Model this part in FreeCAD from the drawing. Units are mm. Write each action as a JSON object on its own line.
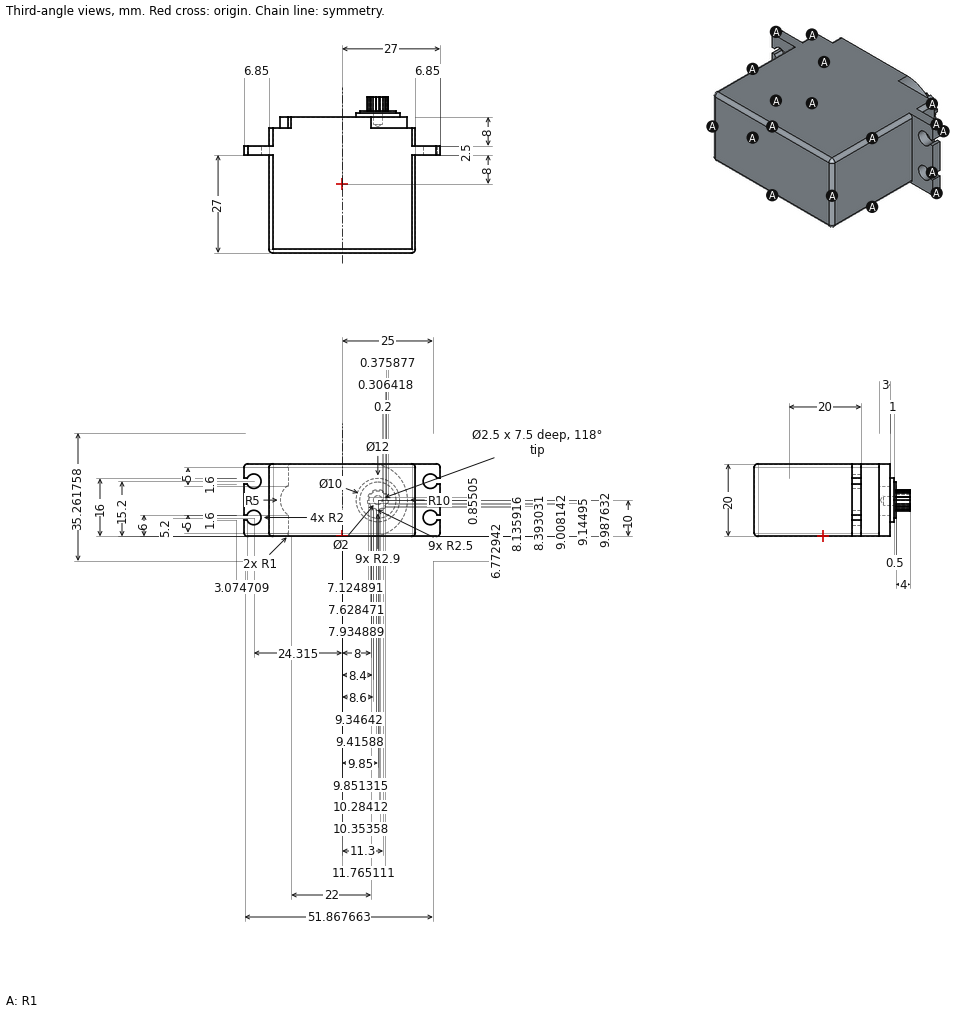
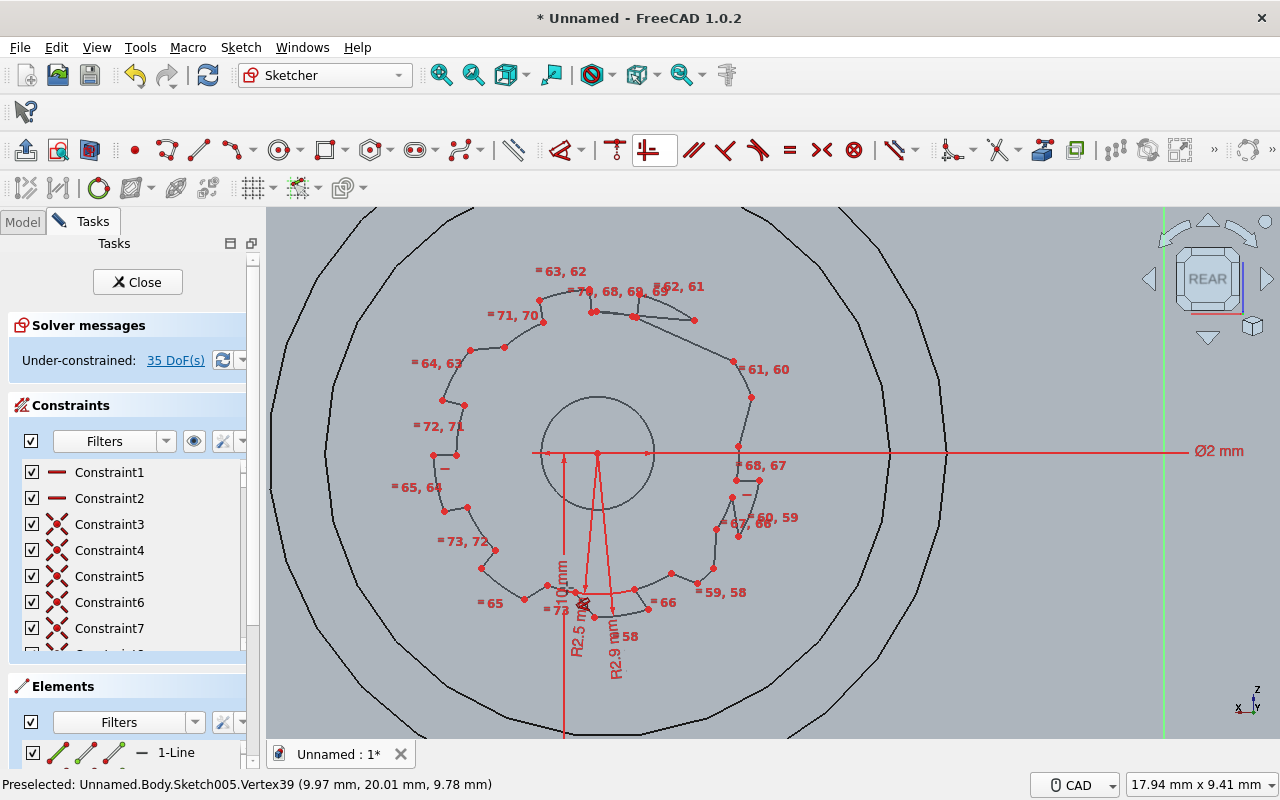
{"action": "left_click", "coordinate": [759, 481]}
{"action": "left_click", "coordinate": [725, 596]}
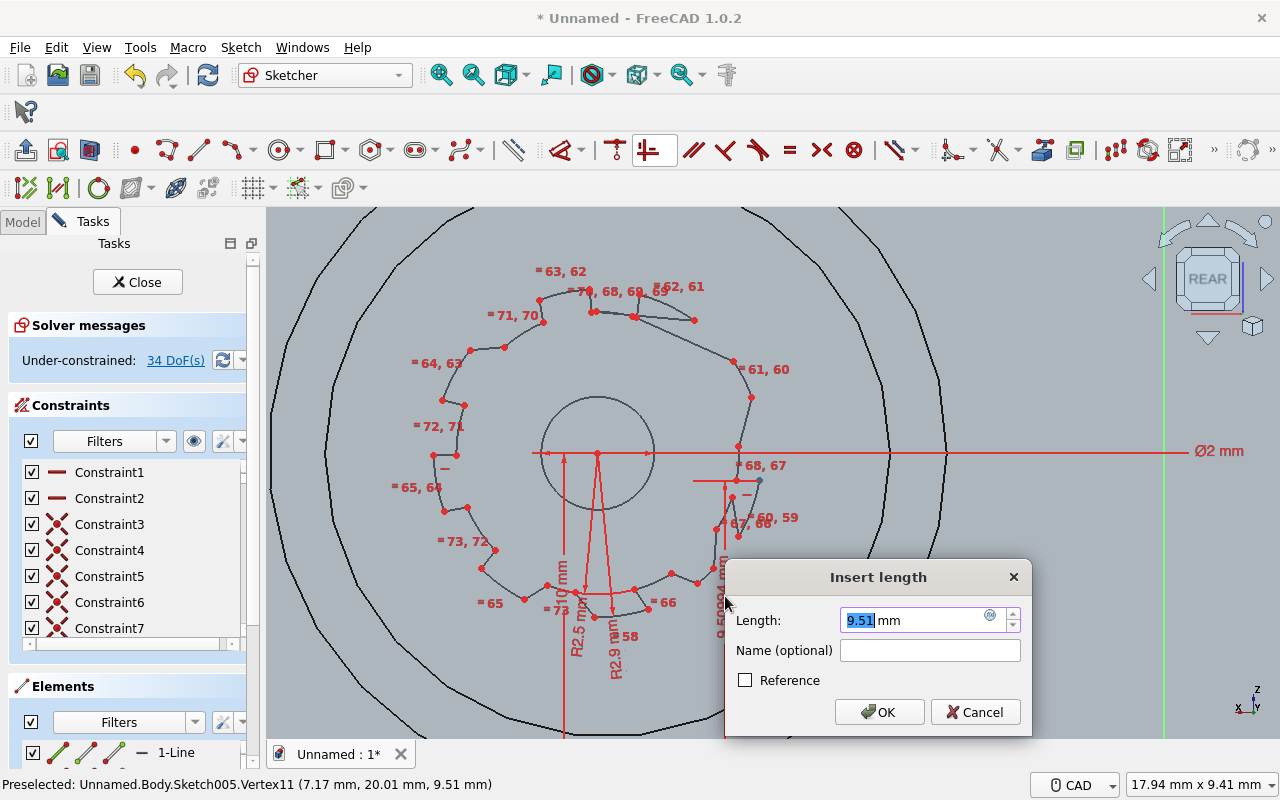
{"action": "type", "text": "10"}
{"action": "key", "text": "Return"}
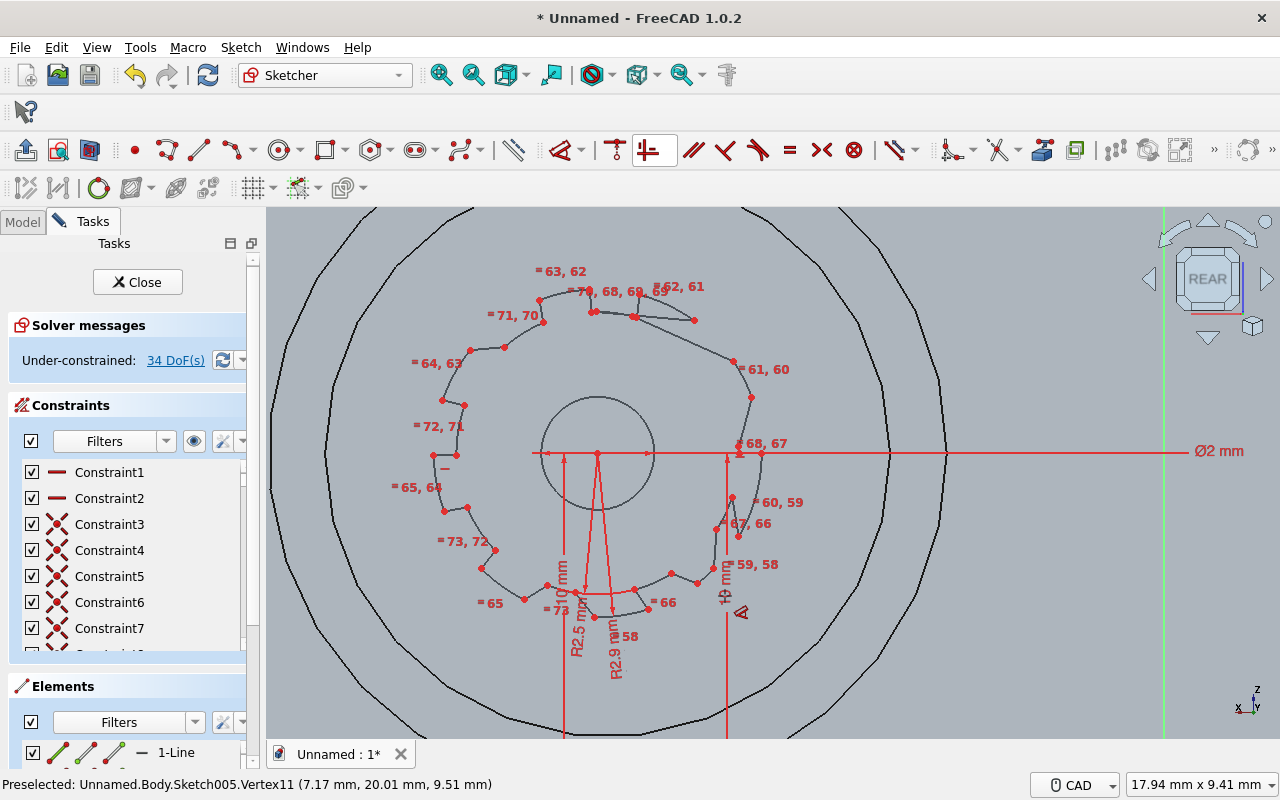
{"action": "left_click", "coordinate": [456, 455]}
{"action": "left_click", "coordinate": [422, 583]}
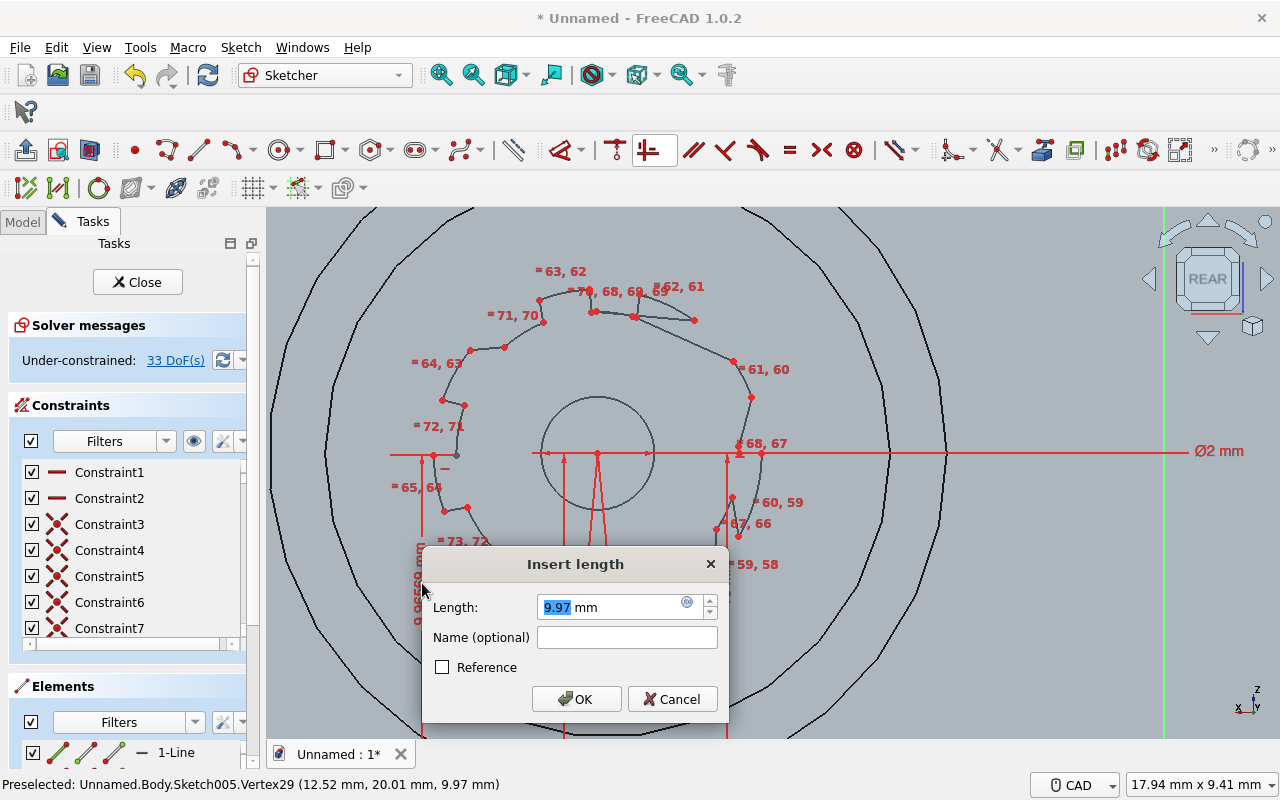
{"action": "type", "text": "10"}
{"action": "key", "text": "Return"}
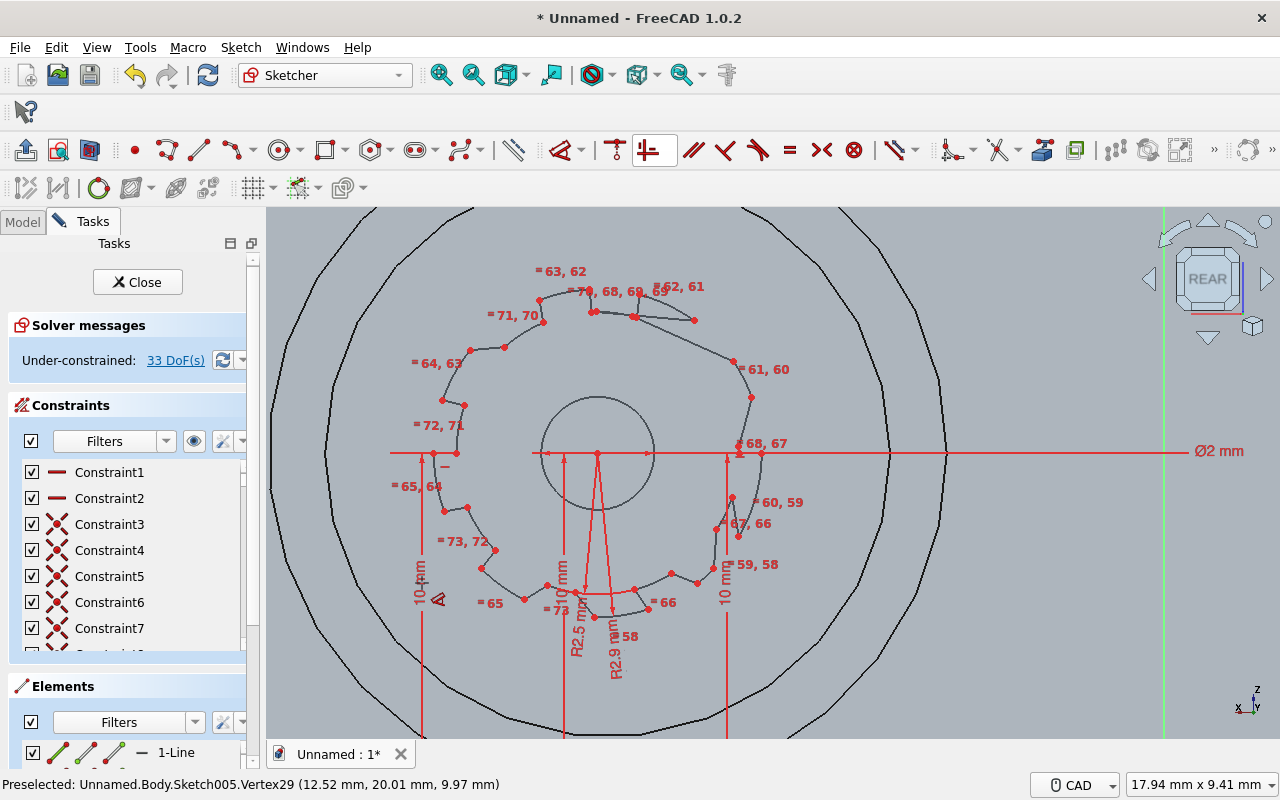
{"action": "left_click", "coordinate": [672, 574]}
{"action": "left_click", "coordinate": [893, 540]}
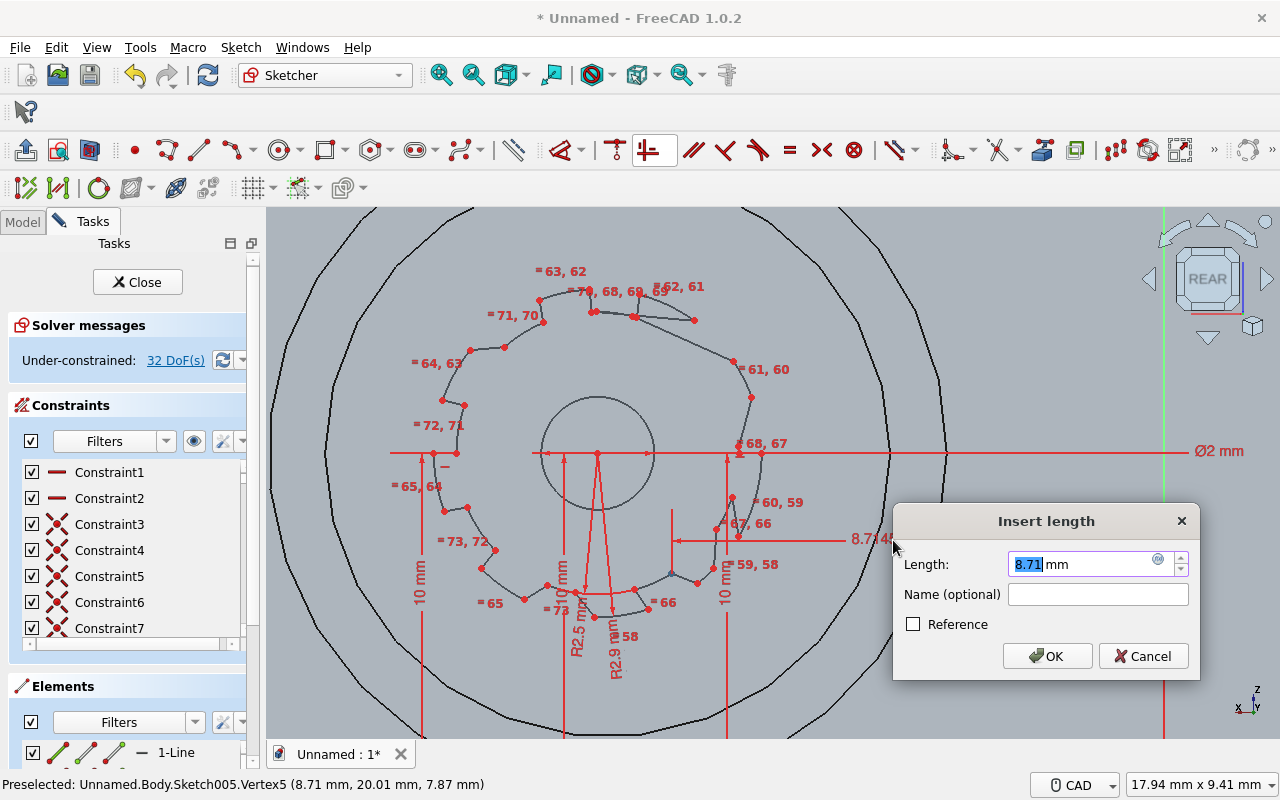
{"action": "type", "text": "8.6"}
{"action": "key", "text": "Return"}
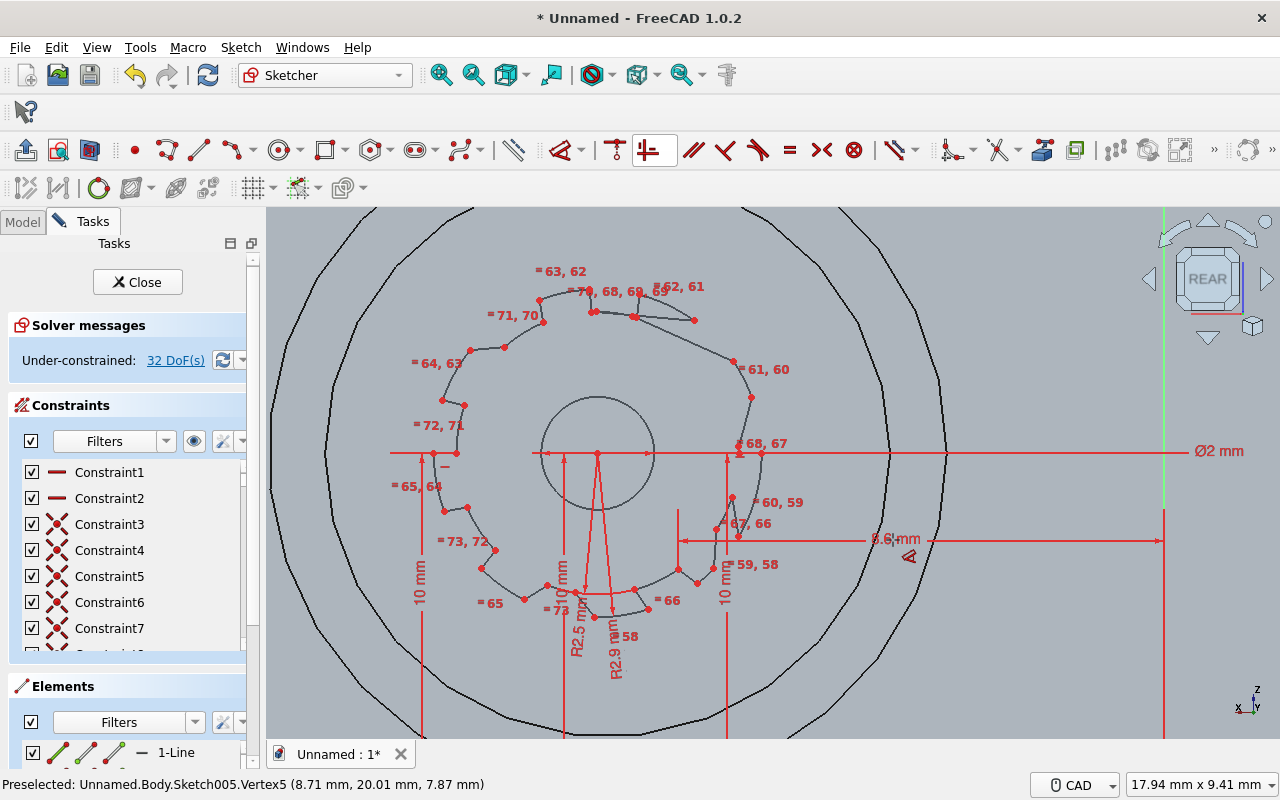
{"action": "left_click", "coordinate": [697, 584]}
{"action": "left_click", "coordinate": [810, 550]}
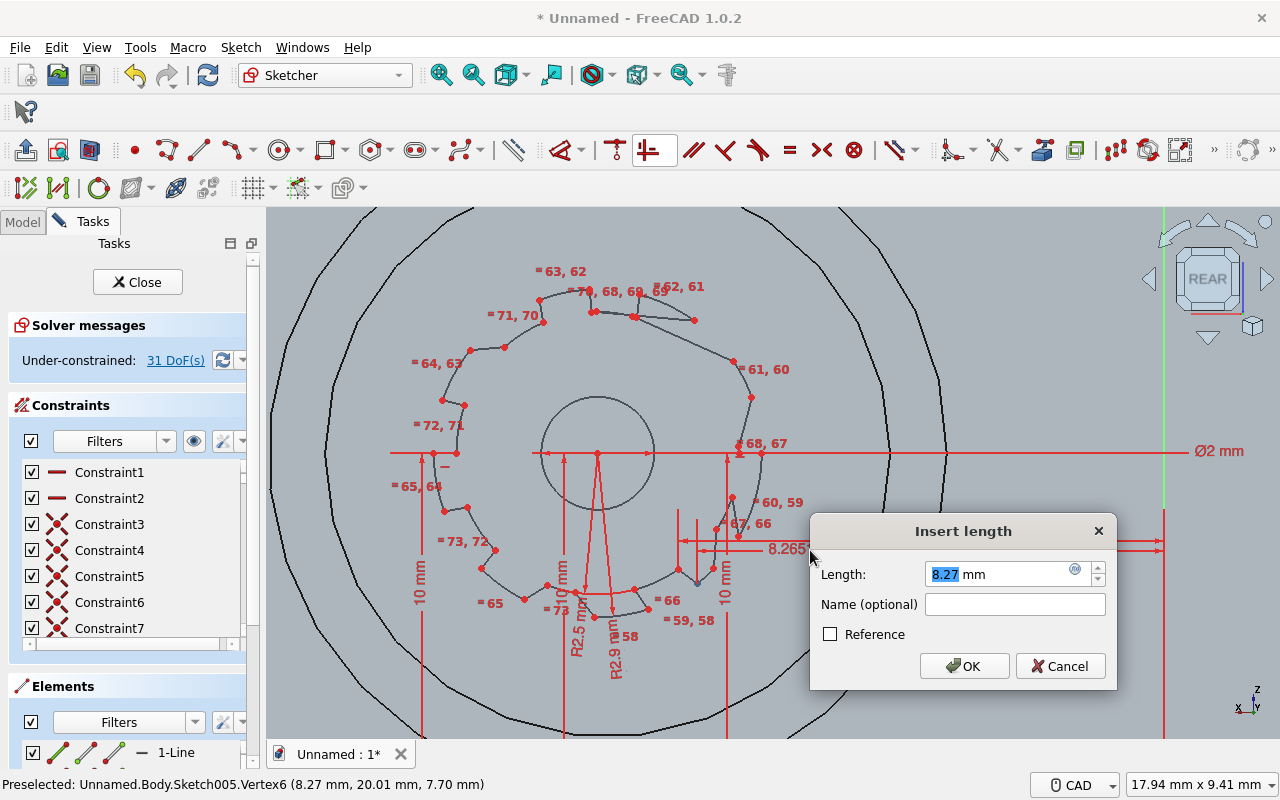
{"action": "type", "text": "8.4"}
{"action": "key", "text": "Return"}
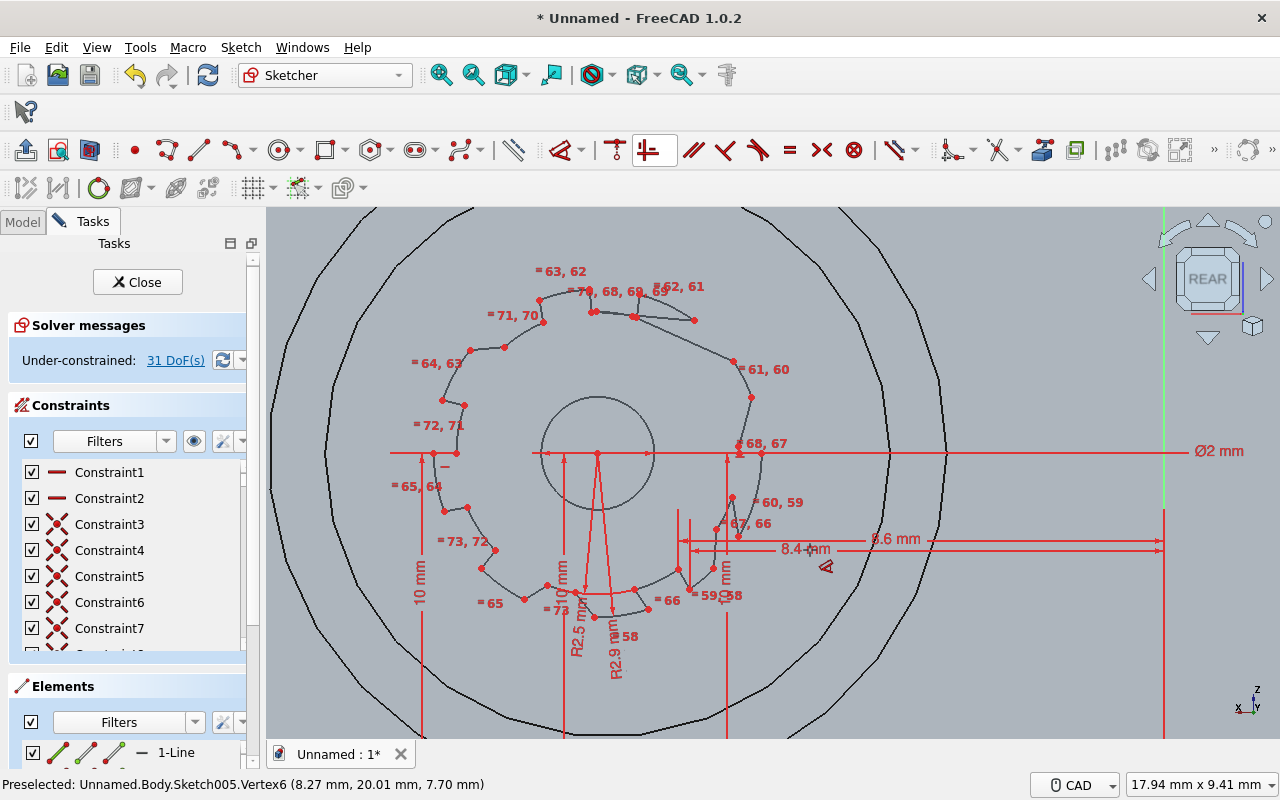
{"action": "scroll", "coordinate": [596, 312], "scroll_direction": "up", "scroll_amount": 5}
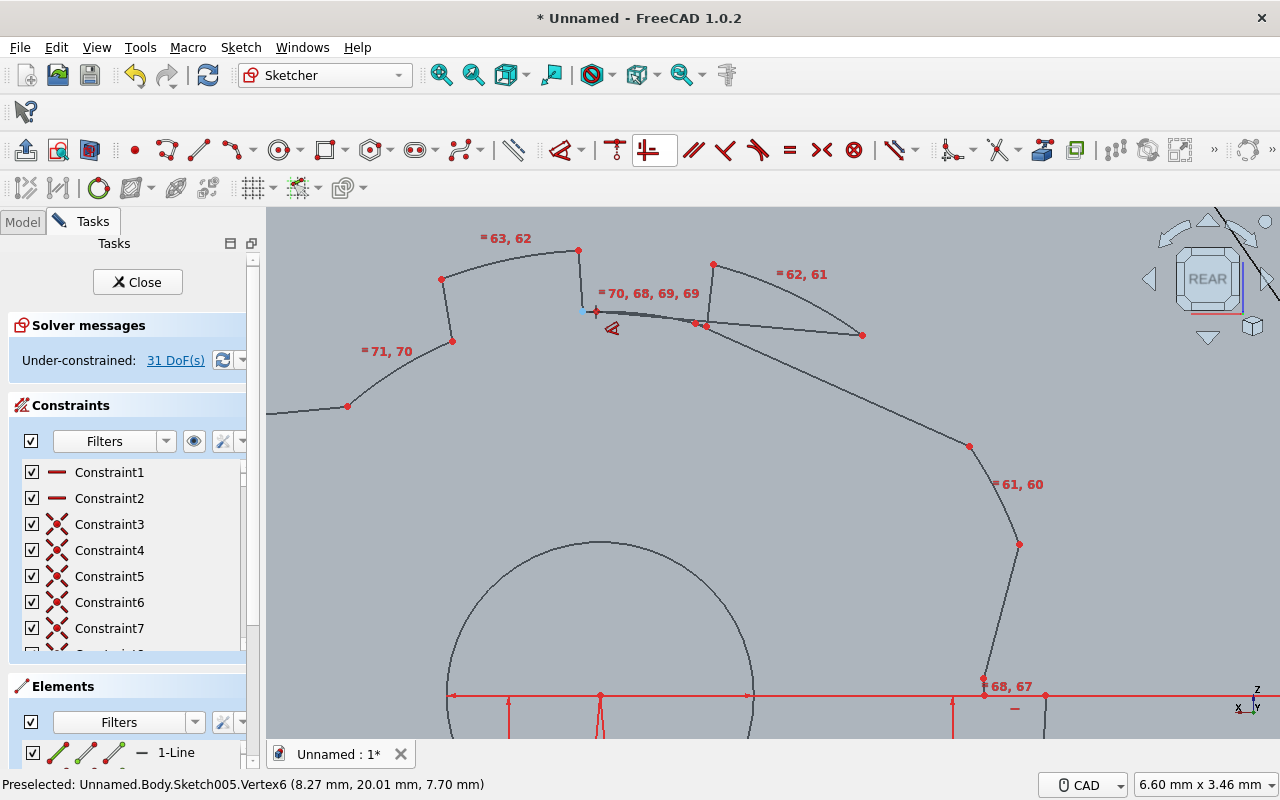
{"action": "left_click", "coordinate": [597, 312]}
{"action": "left_click", "coordinate": [856, 278]}